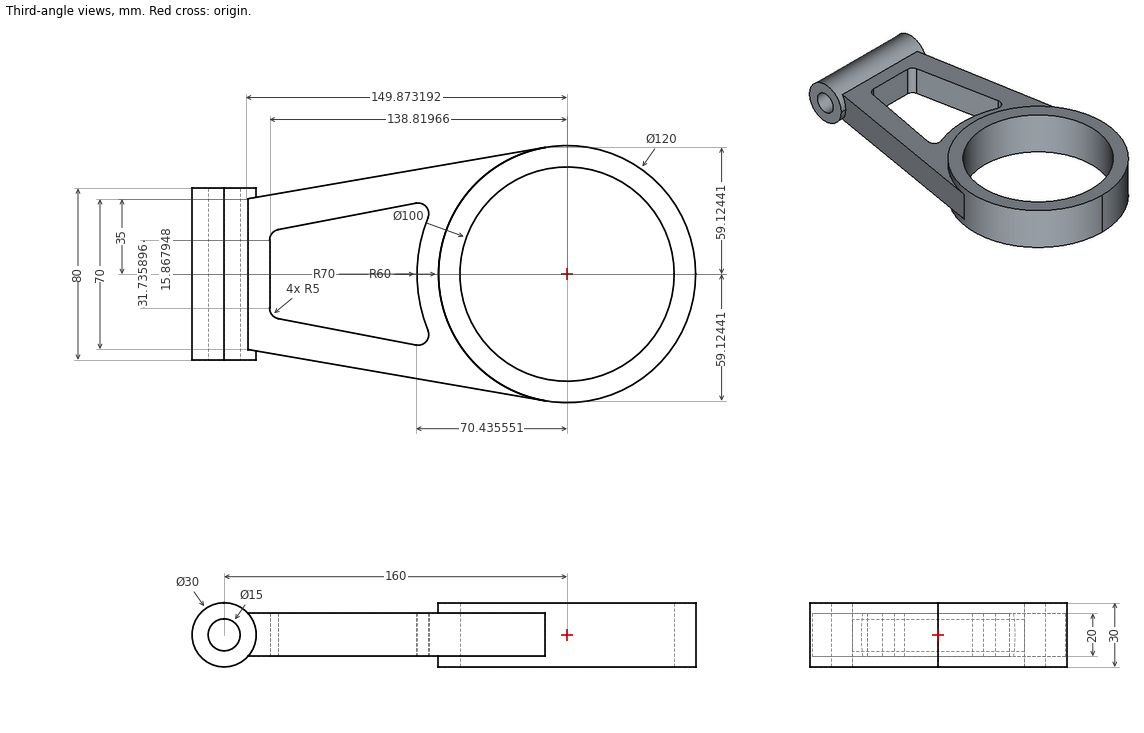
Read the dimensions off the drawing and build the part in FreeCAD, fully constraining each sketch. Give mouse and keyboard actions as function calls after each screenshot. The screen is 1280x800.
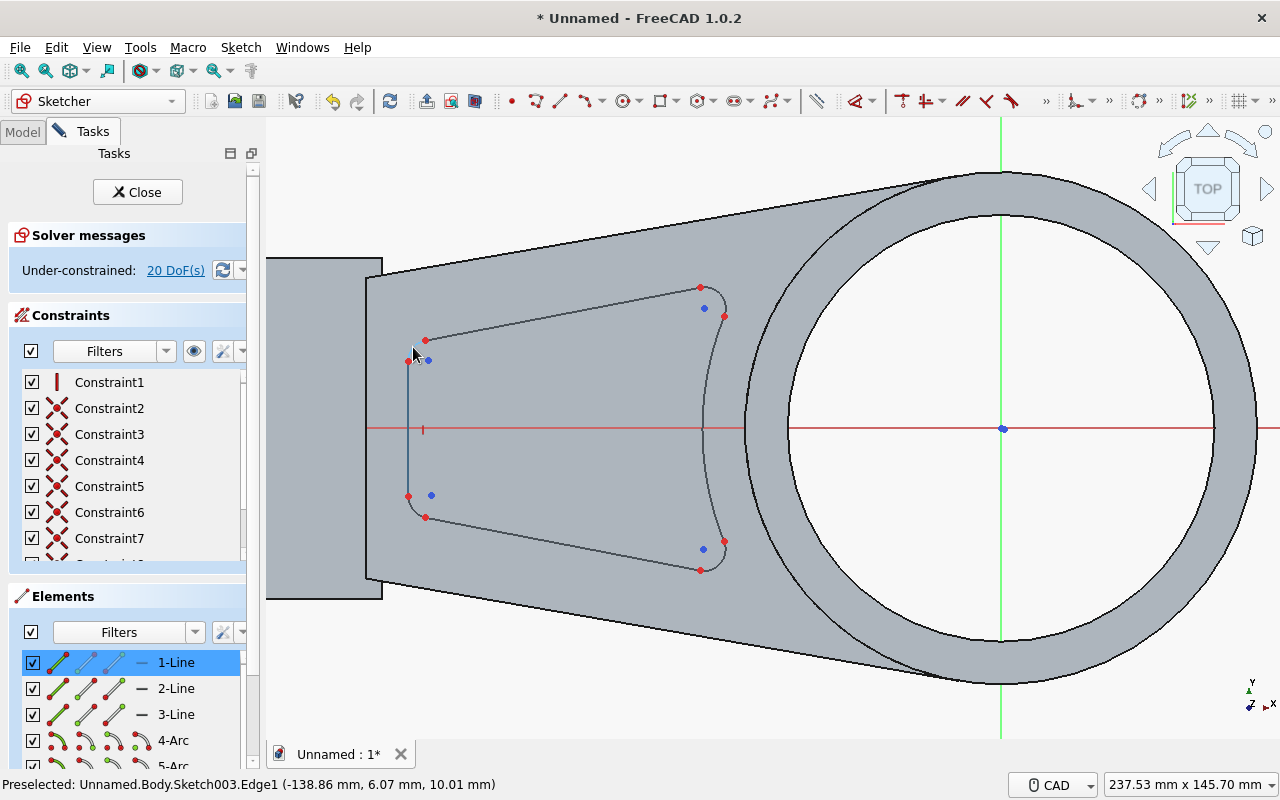
scroll(410, 505, up, 3)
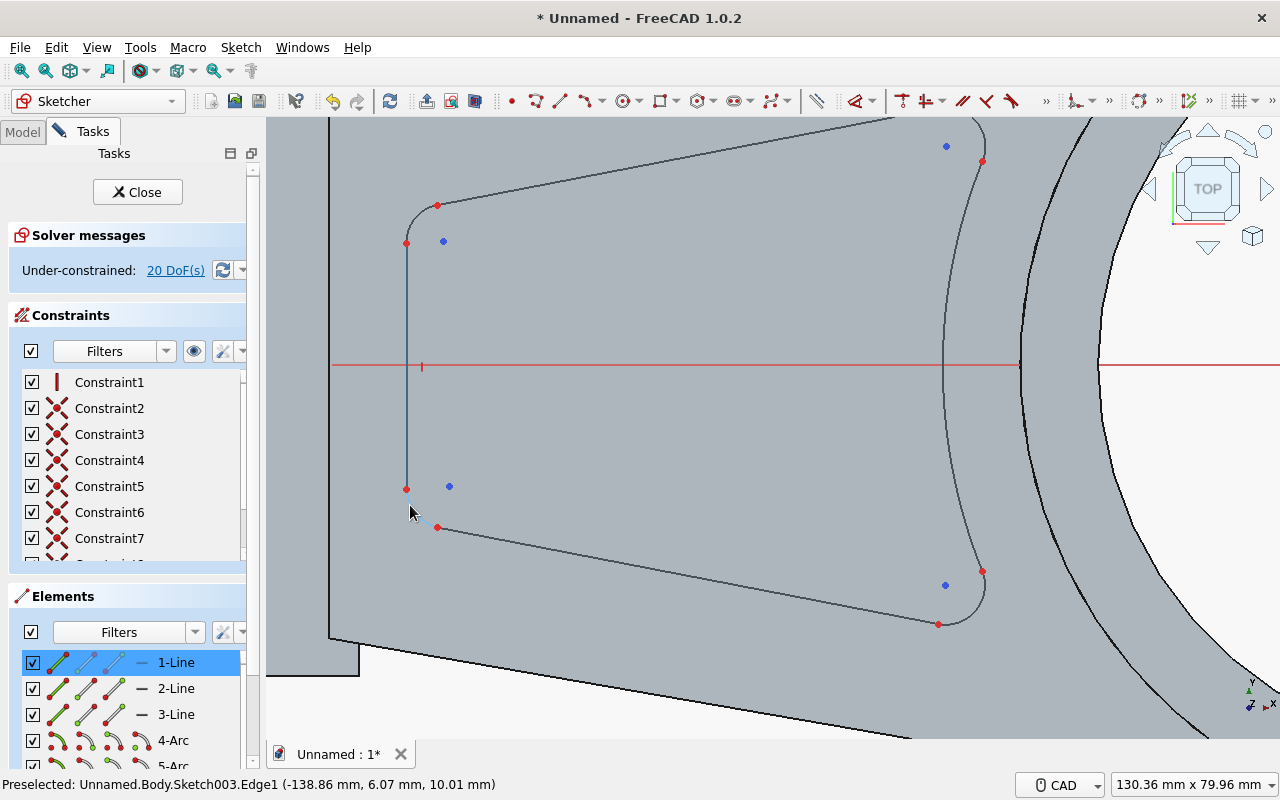
click(411, 505)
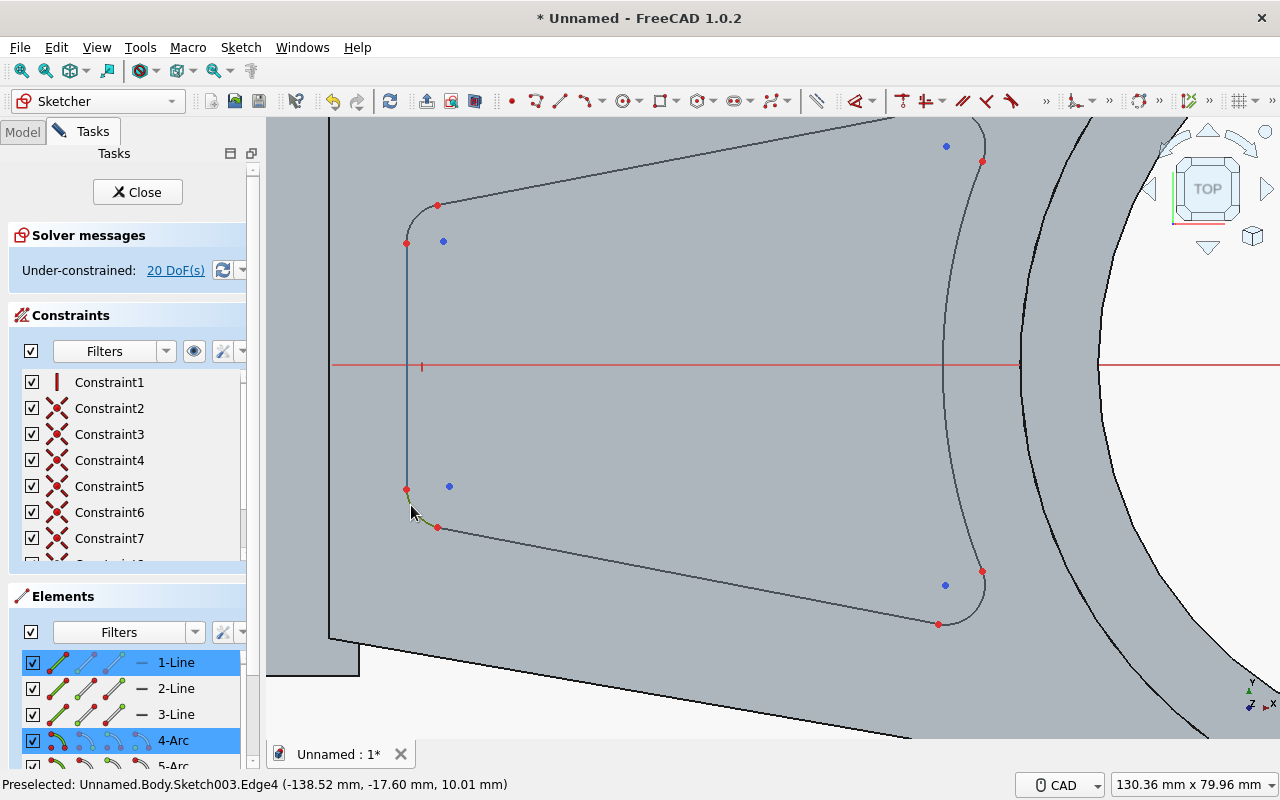
click(1012, 102)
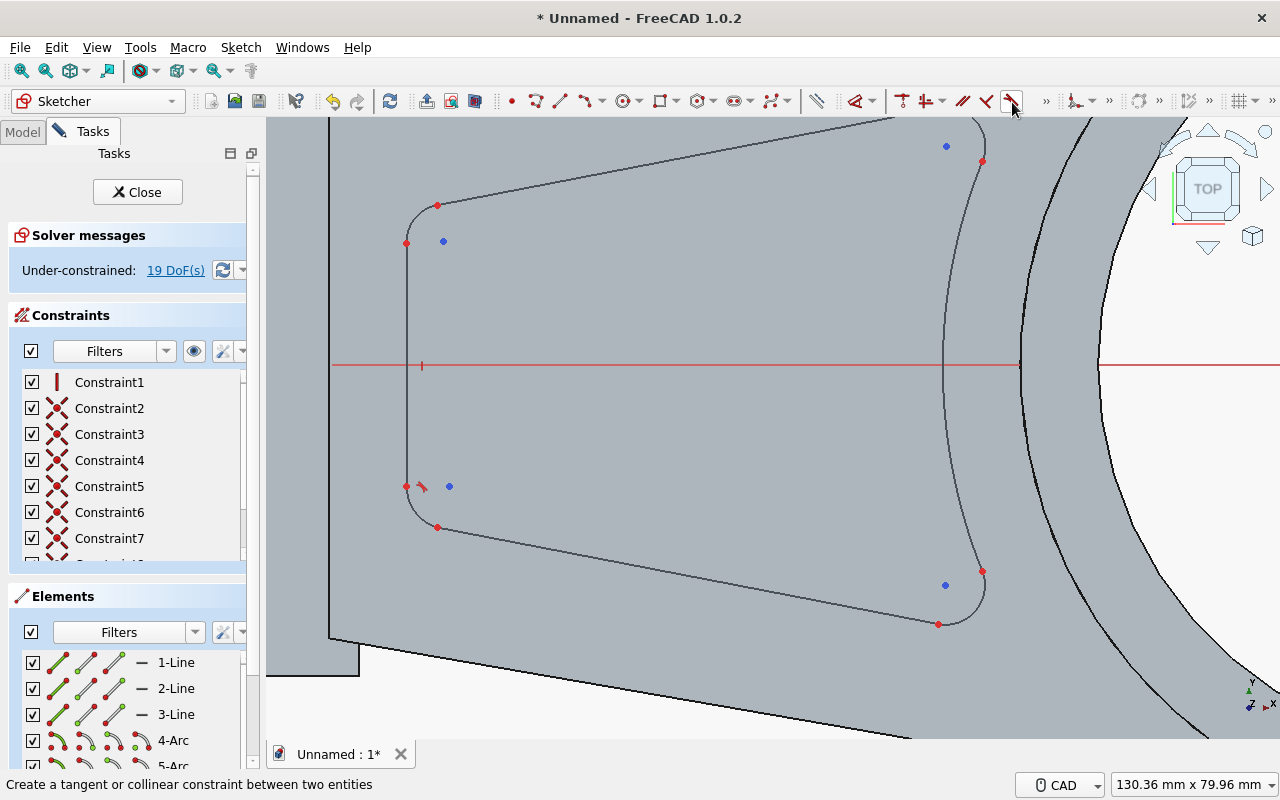
click(407, 316)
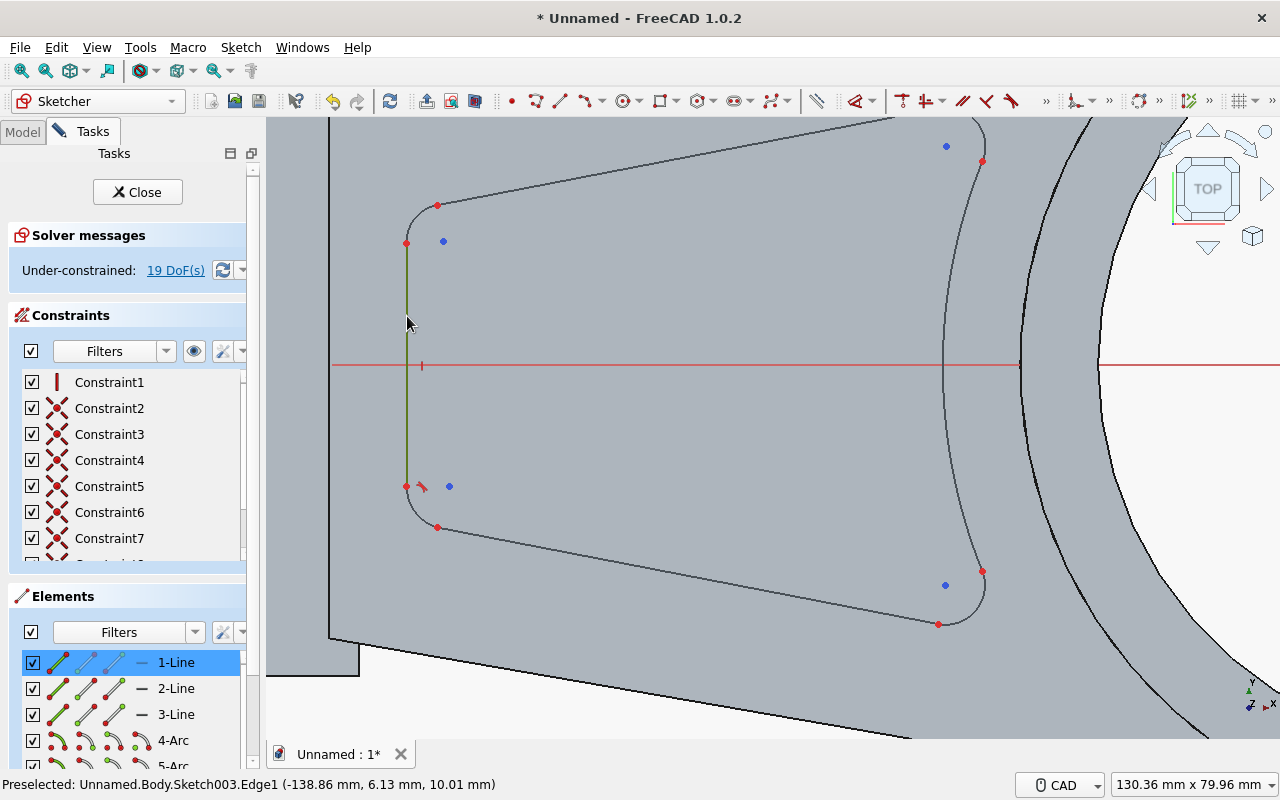
click(423, 211)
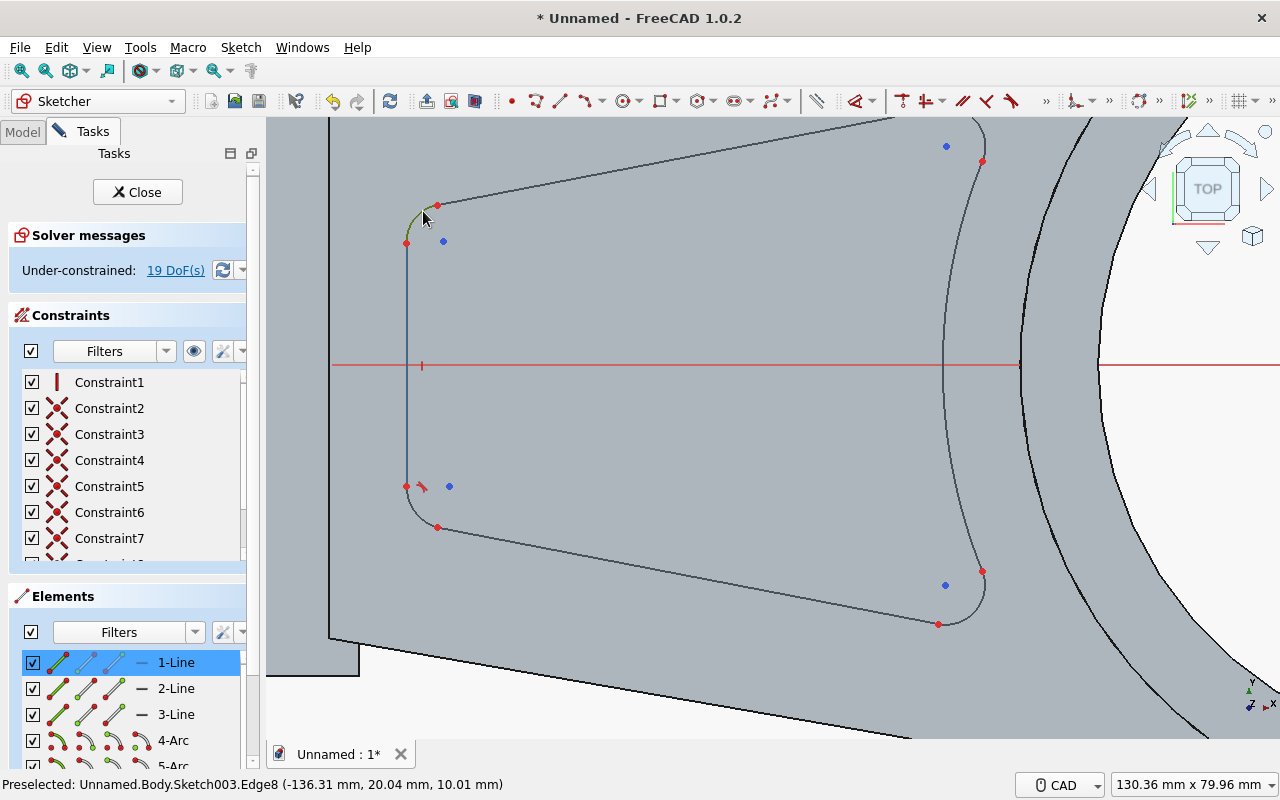
click(1012, 102)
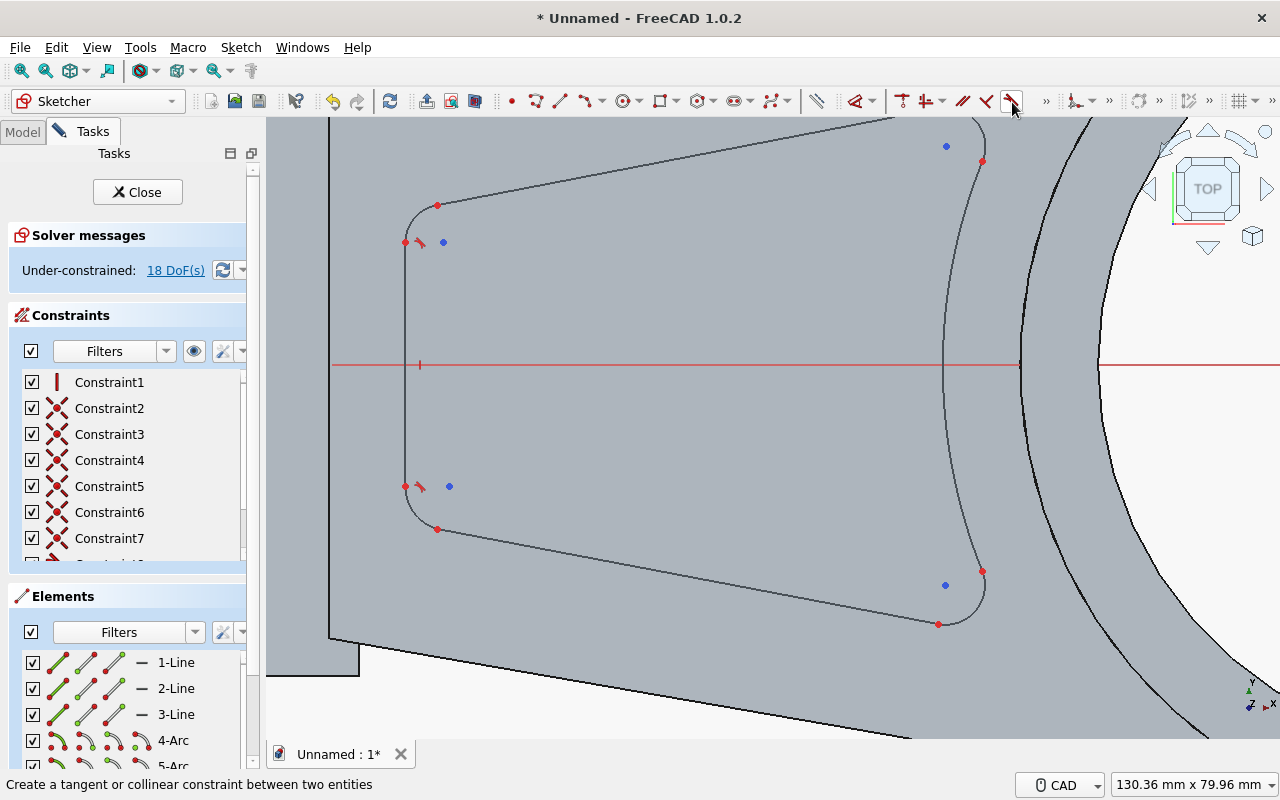
click(588, 558)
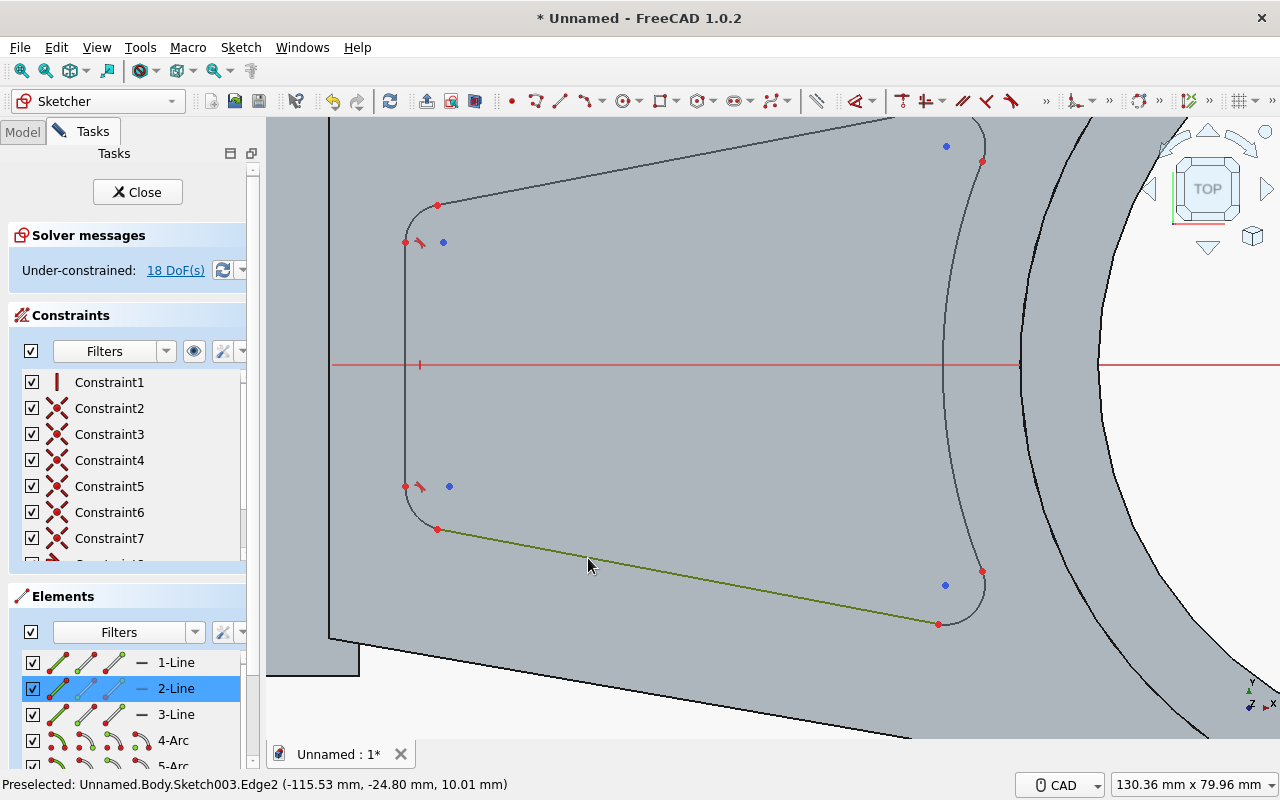
click(409, 503)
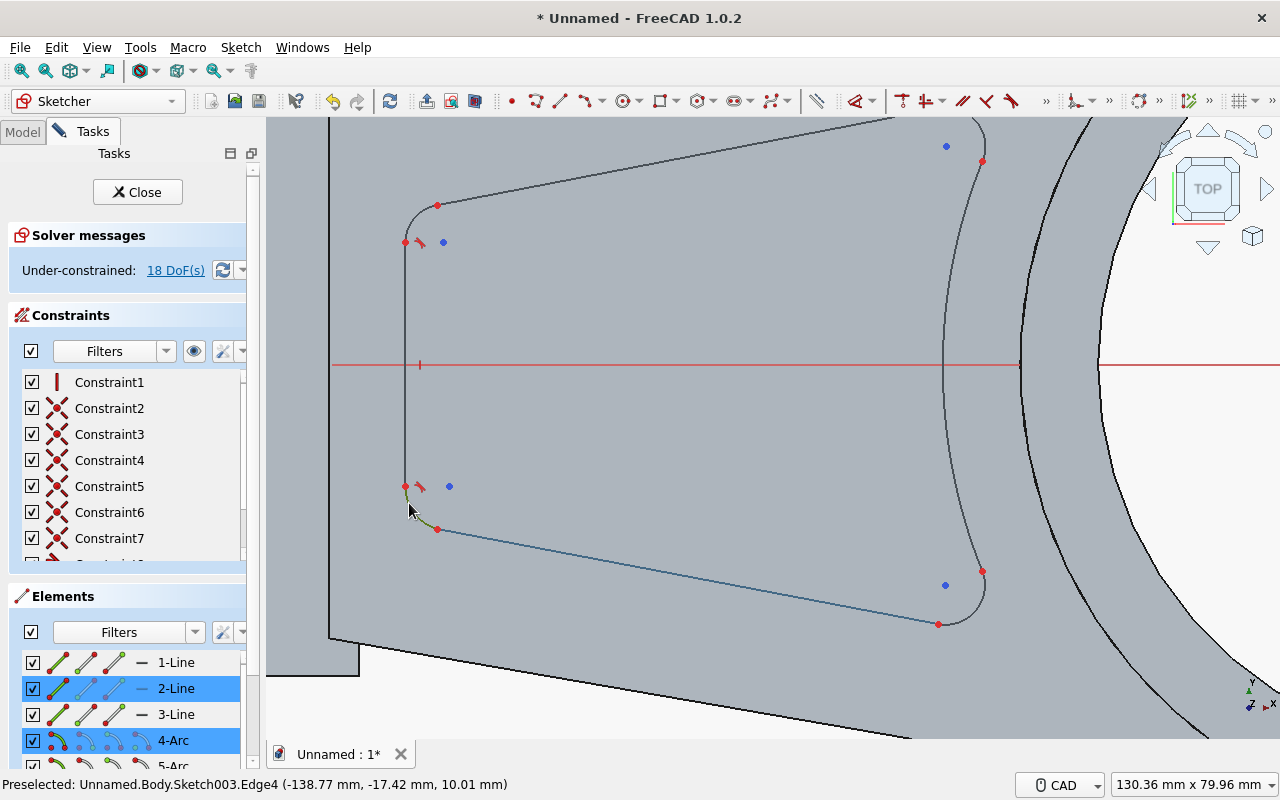
click(1012, 102)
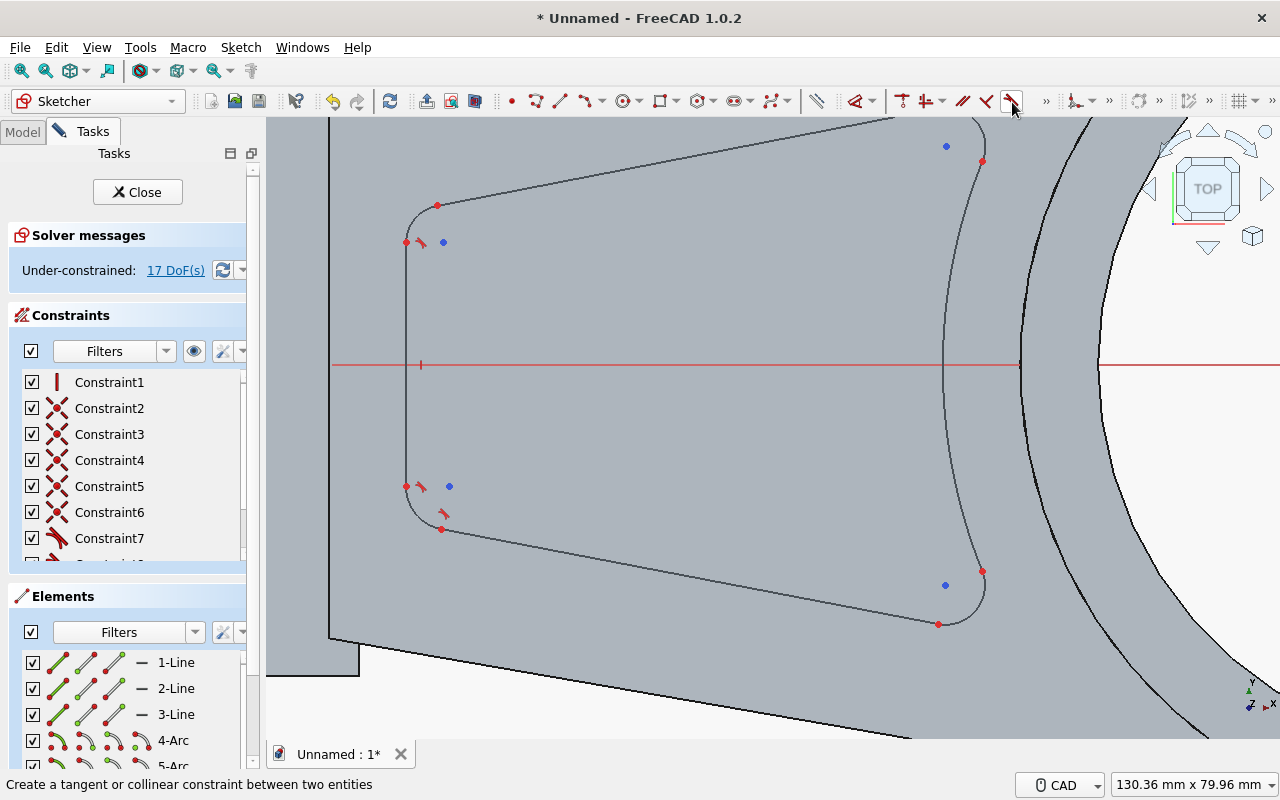
click(590, 558)